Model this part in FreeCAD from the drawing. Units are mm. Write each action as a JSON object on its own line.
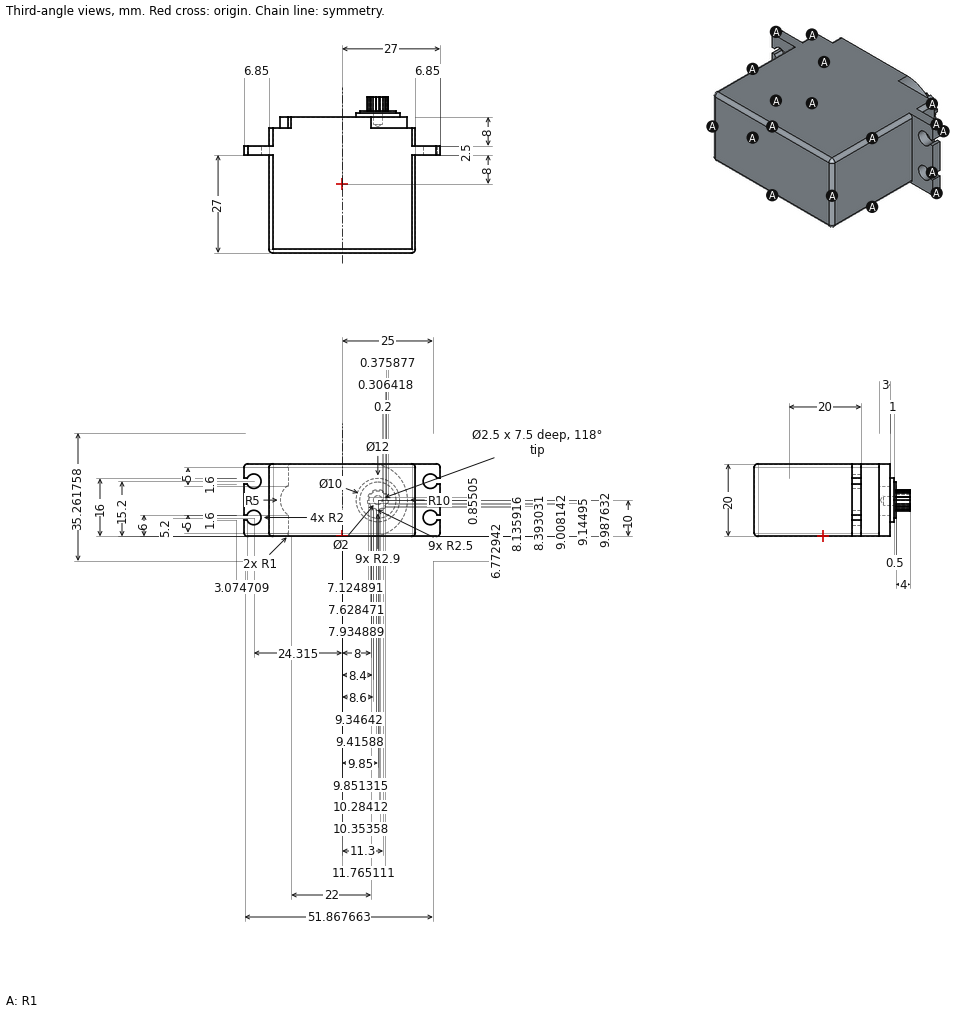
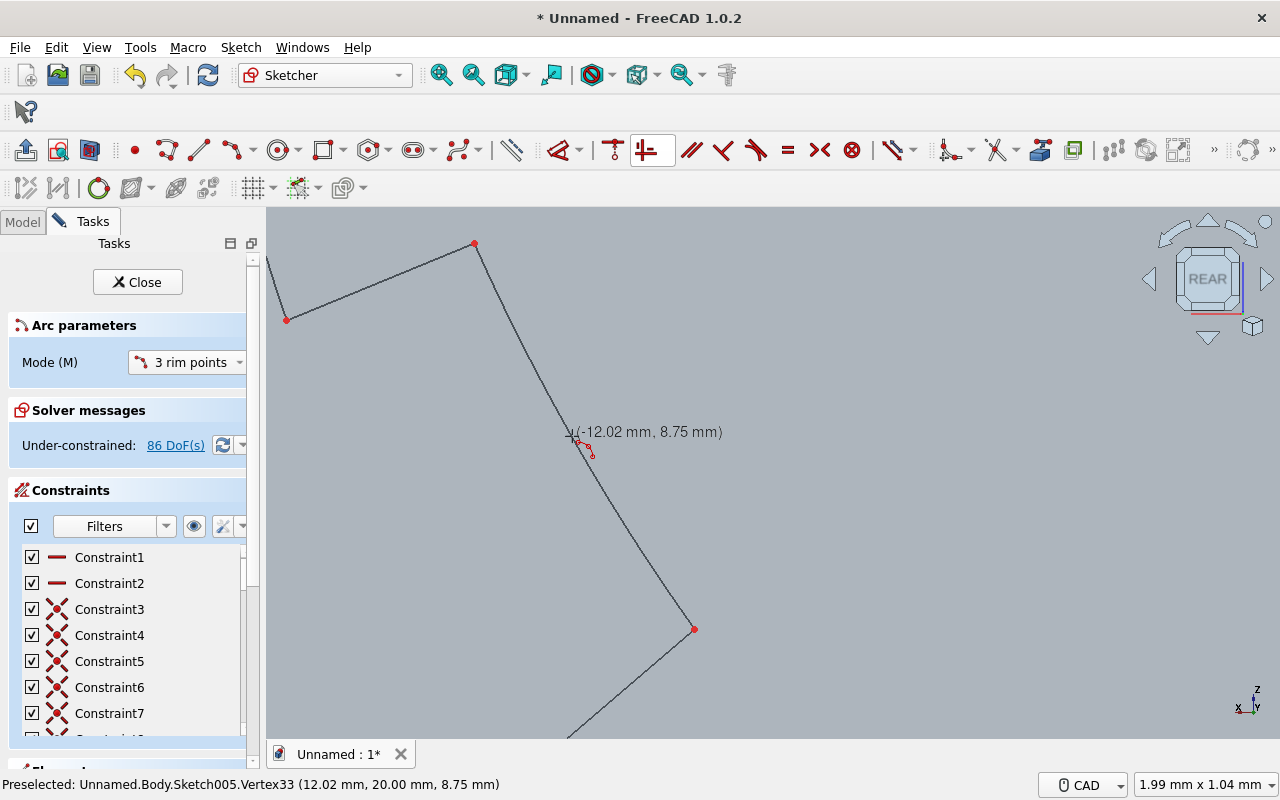
{"action": "scroll", "coordinate": [561, 413], "scroll_direction": "down", "scroll_amount": 15}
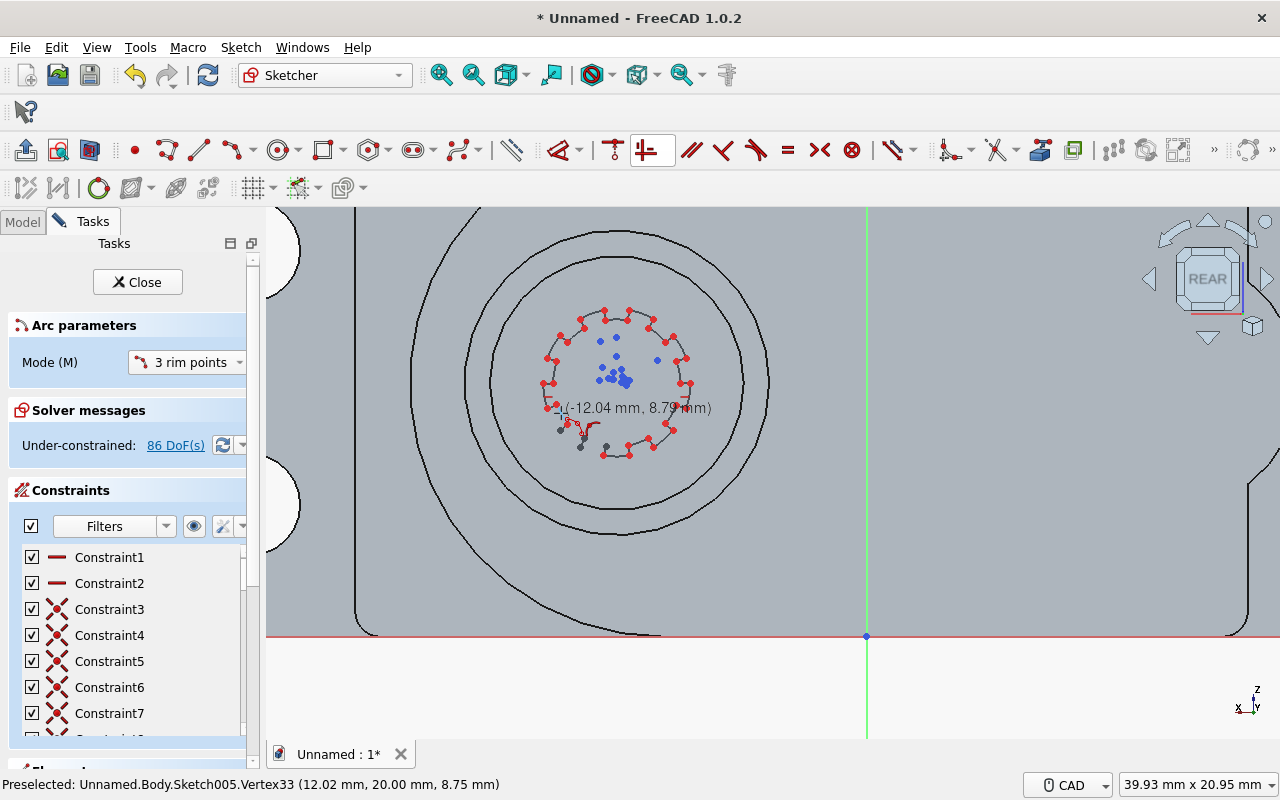
{"action": "scroll", "coordinate": [560, 430], "scroll_direction": "up", "scroll_amount": 6}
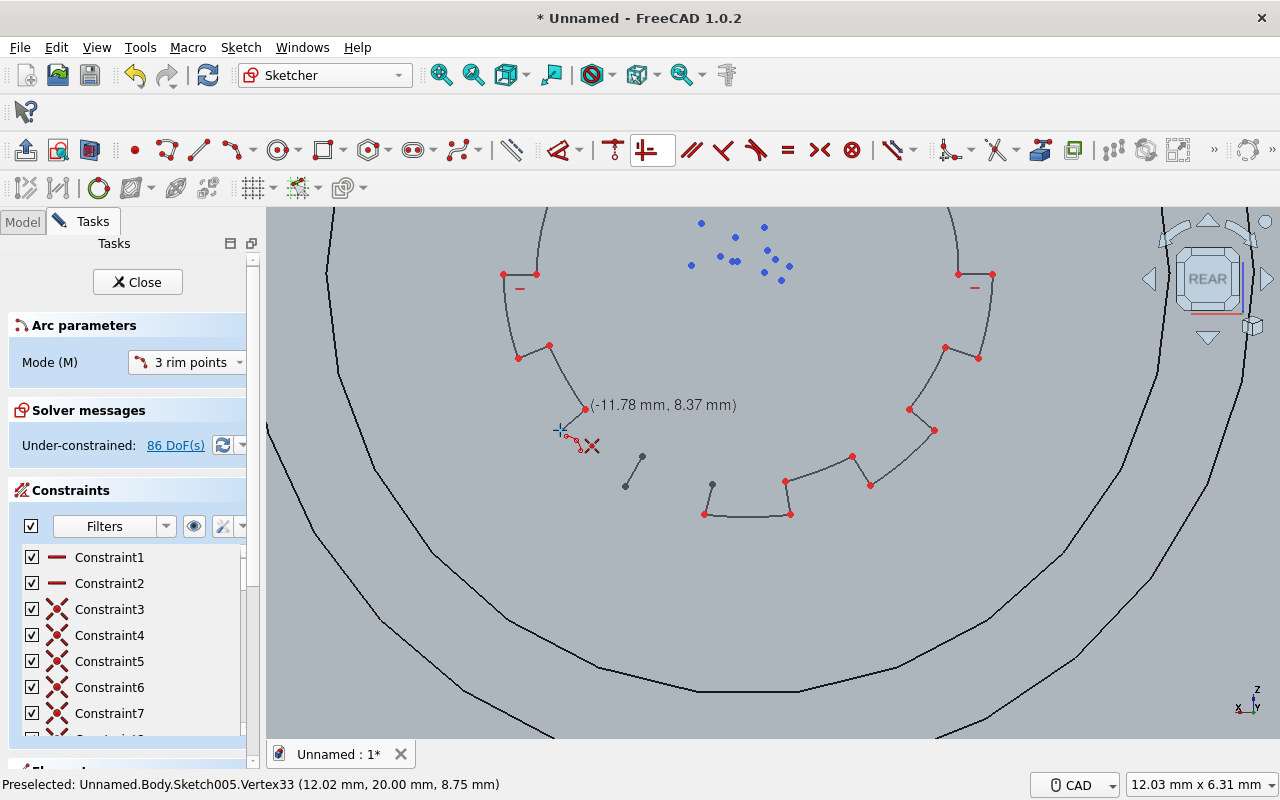
{"action": "left_click", "coordinate": [560, 431]}
{"action": "left_click", "coordinate": [626, 486]}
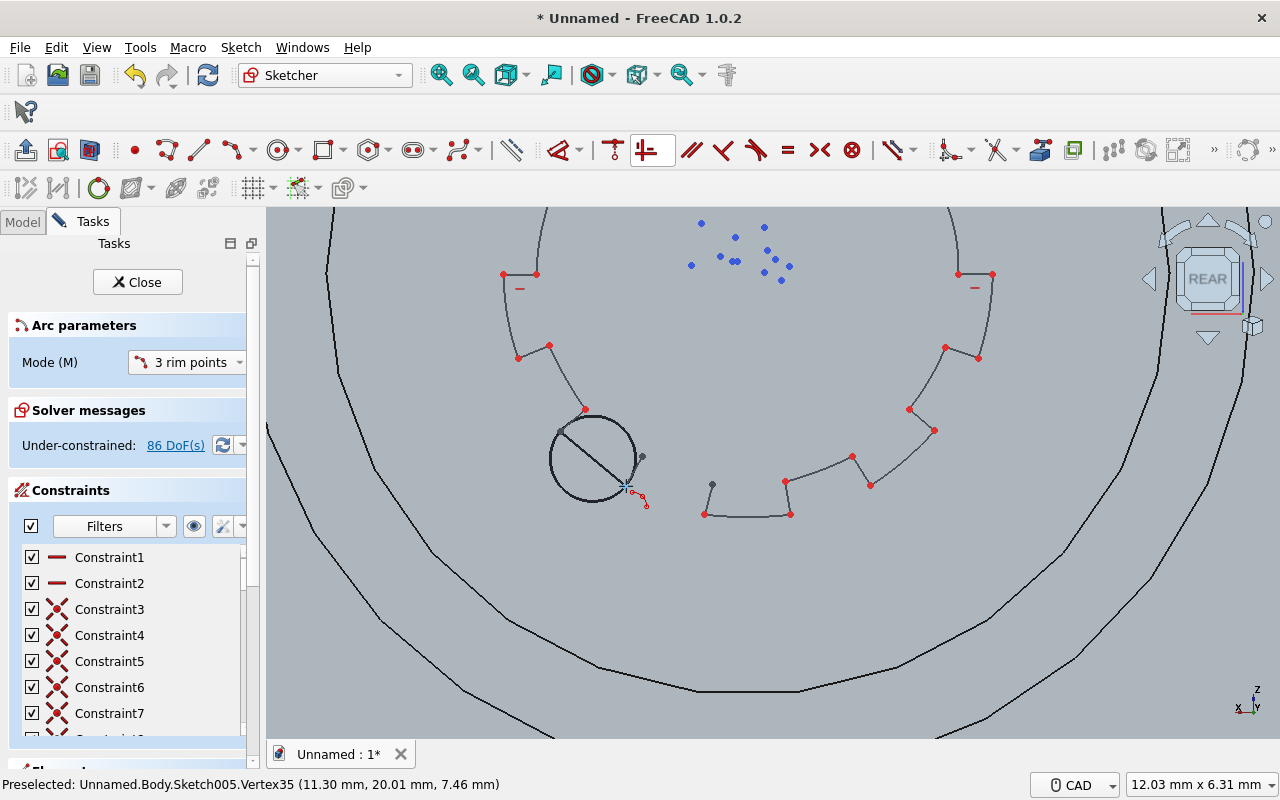
{"action": "scroll", "coordinate": [591, 460], "scroll_direction": "up", "scroll_amount": 8}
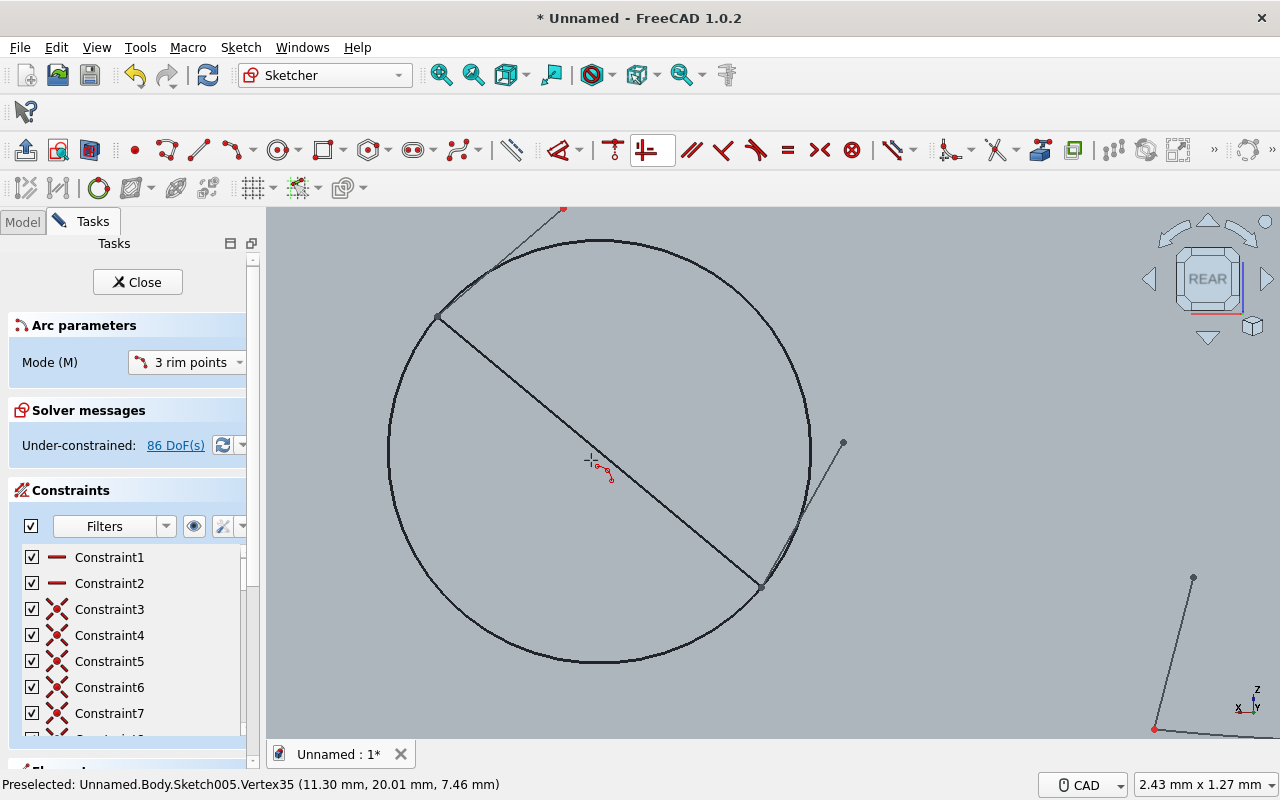
{"action": "left_click", "coordinate": [589, 456]}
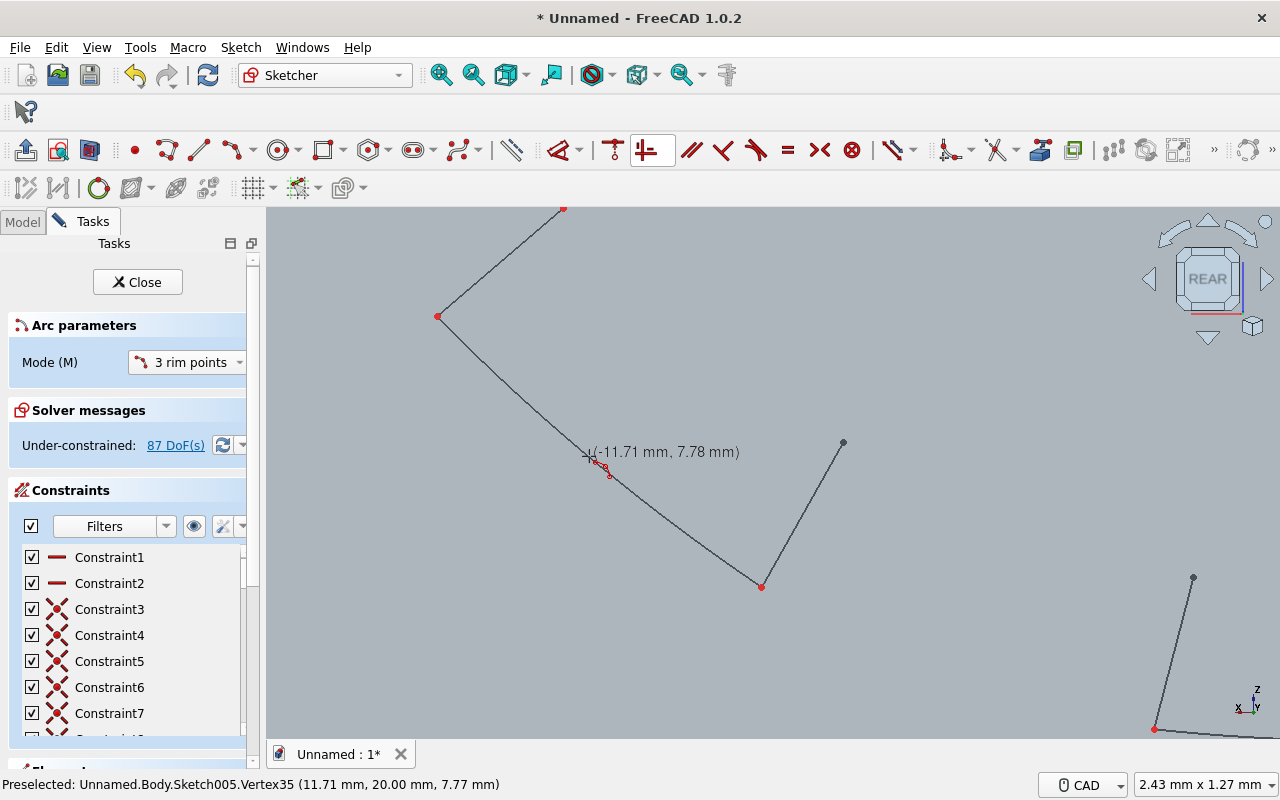
{"action": "scroll", "coordinate": [568, 438], "scroll_direction": "down", "scroll_amount": 14}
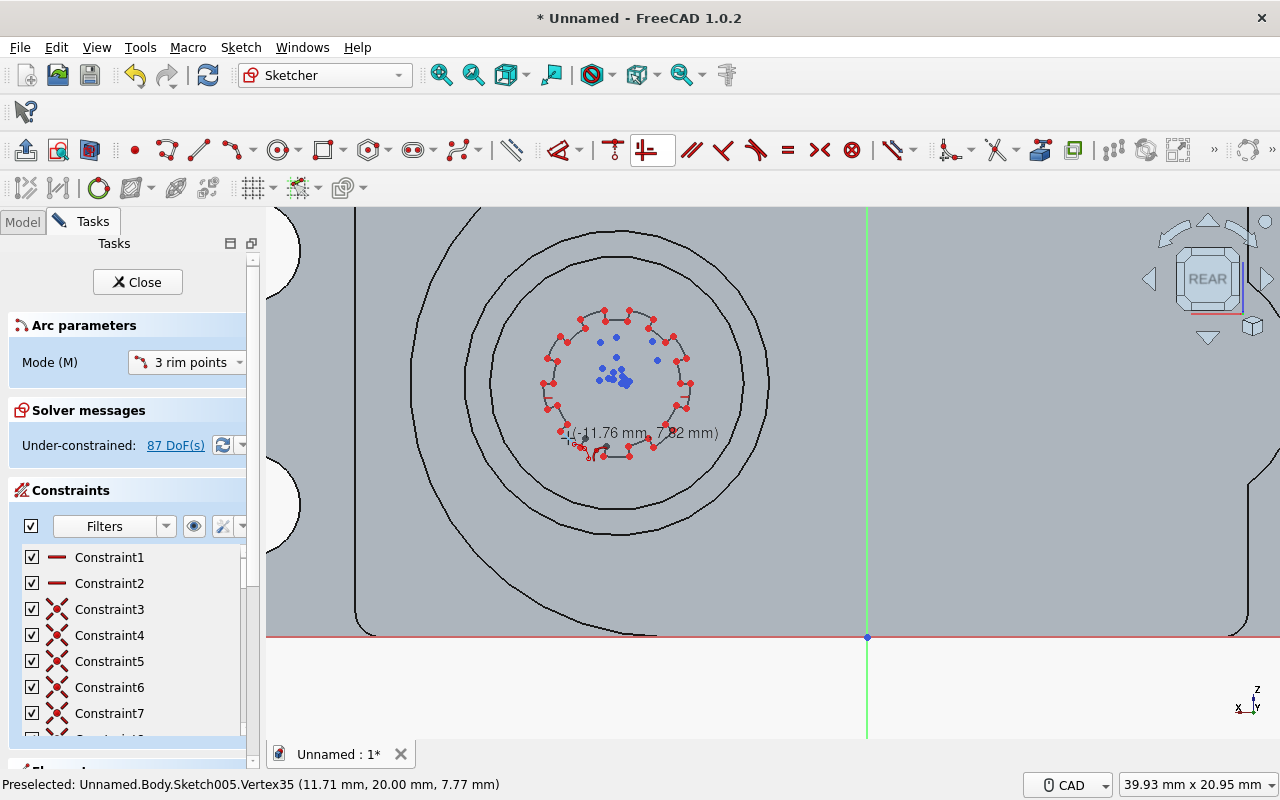
{"action": "scroll", "coordinate": [585, 438], "scroll_direction": "up", "scroll_amount": 6}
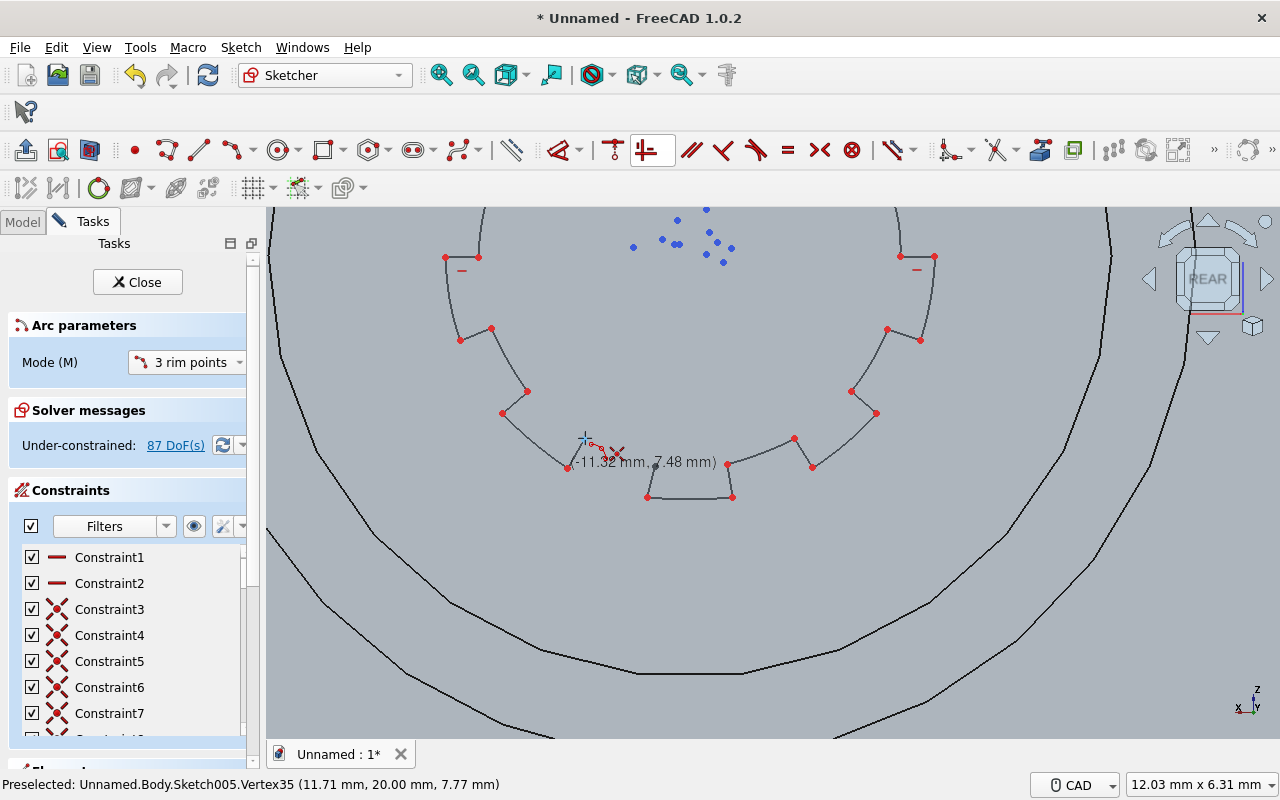
{"action": "left_click", "coordinate": [584, 439]}
{"action": "left_click", "coordinate": [655, 467]}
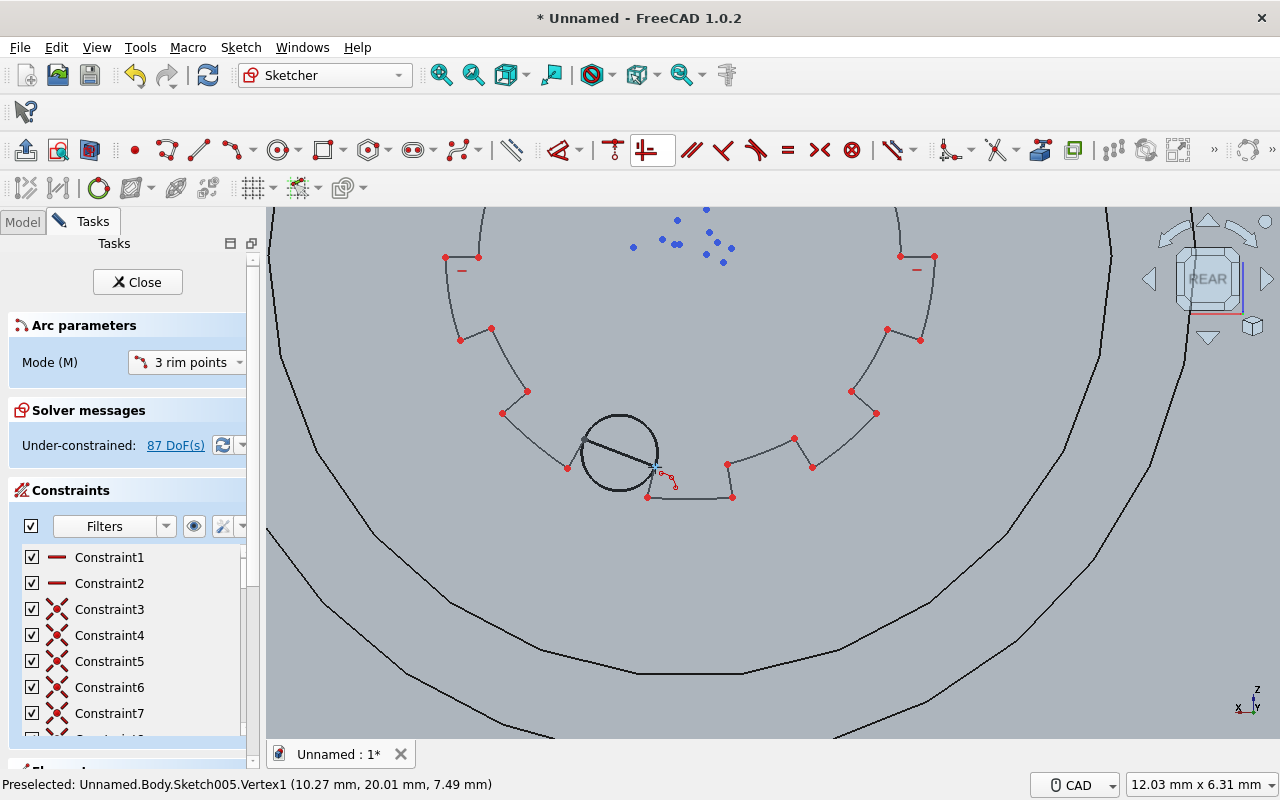
{"action": "scroll", "coordinate": [618, 453], "scroll_direction": "up", "scroll_amount": 9}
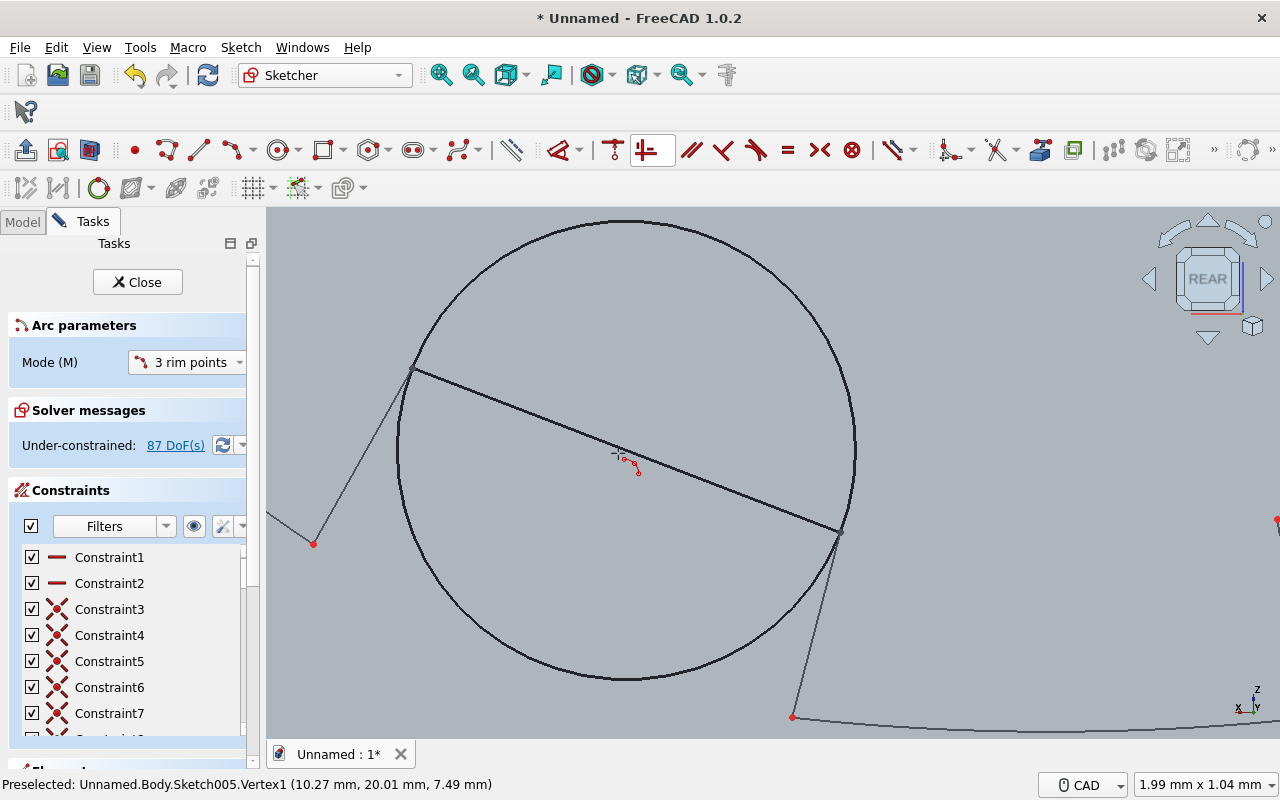
{"action": "left_click", "coordinate": [617, 449]}